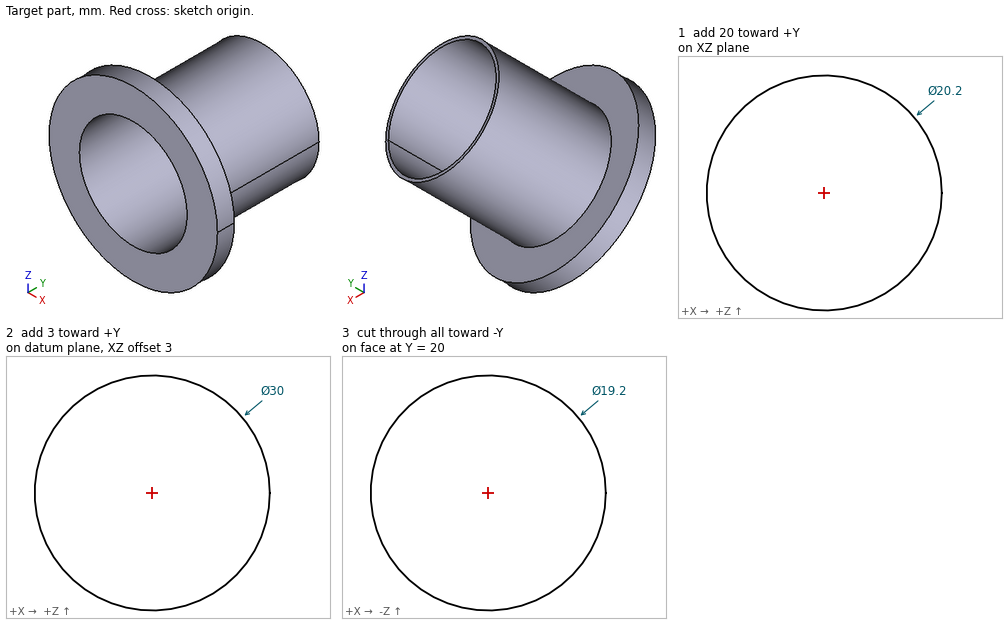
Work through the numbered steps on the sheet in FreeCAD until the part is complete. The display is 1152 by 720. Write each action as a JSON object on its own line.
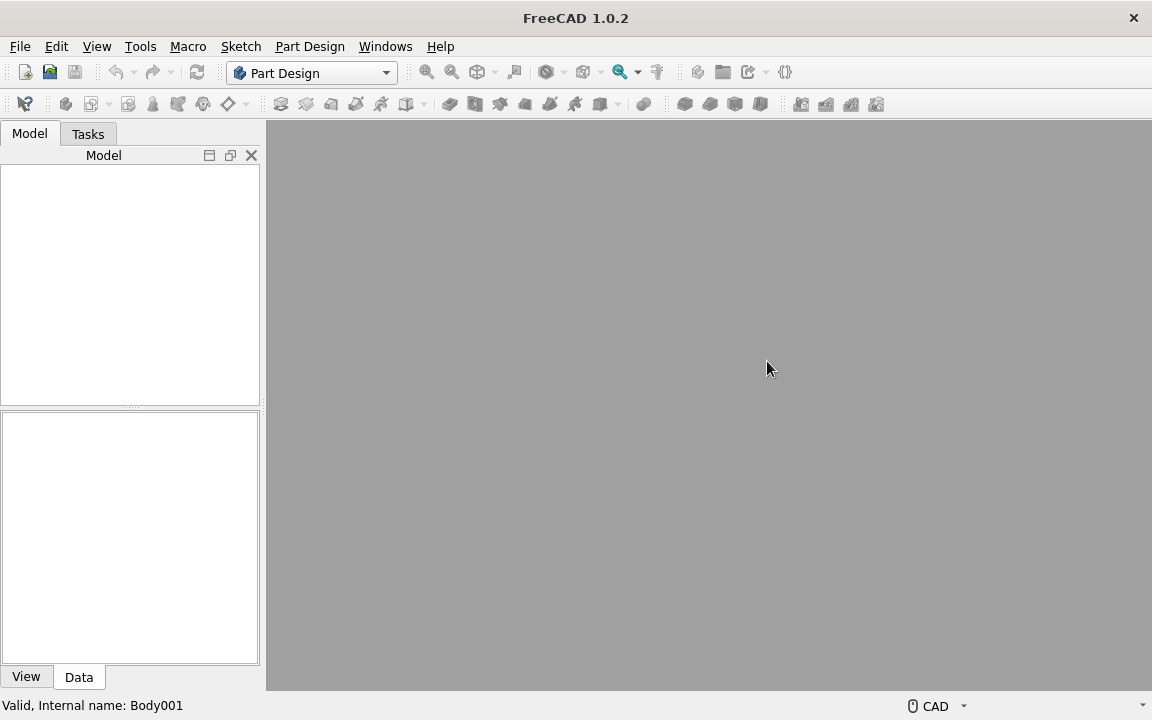
{"action": "key", "text": "ctrl+n"}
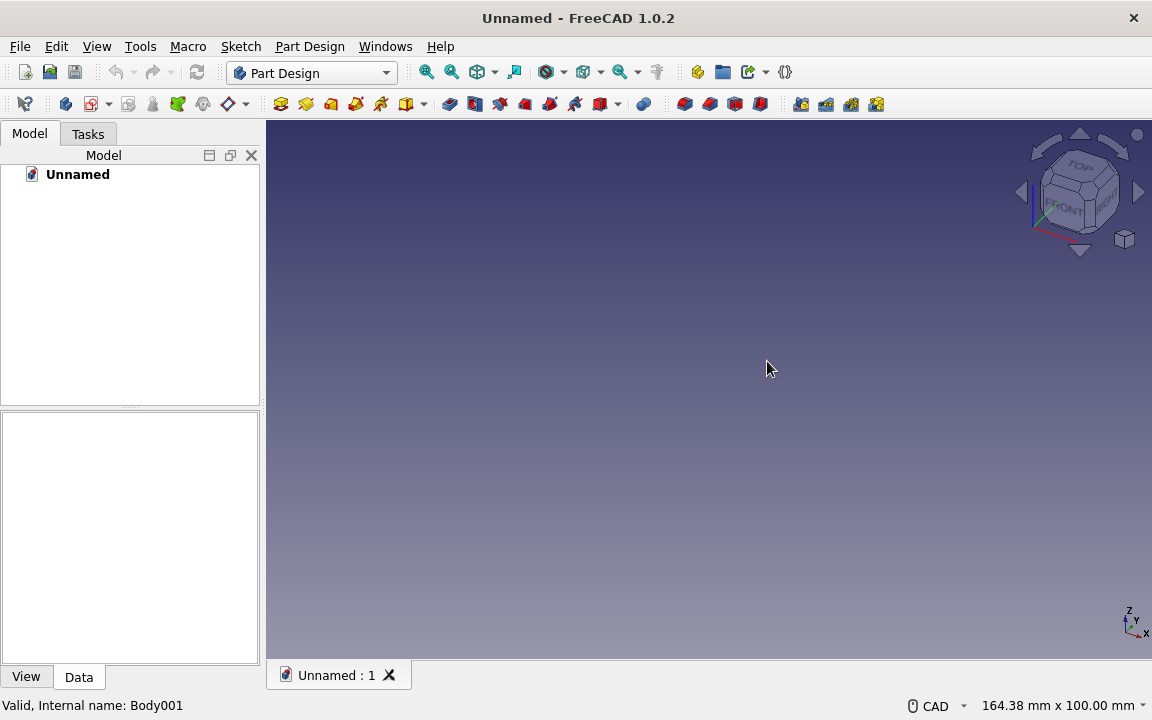
{"action": "left_click", "coordinate": [90, 104]}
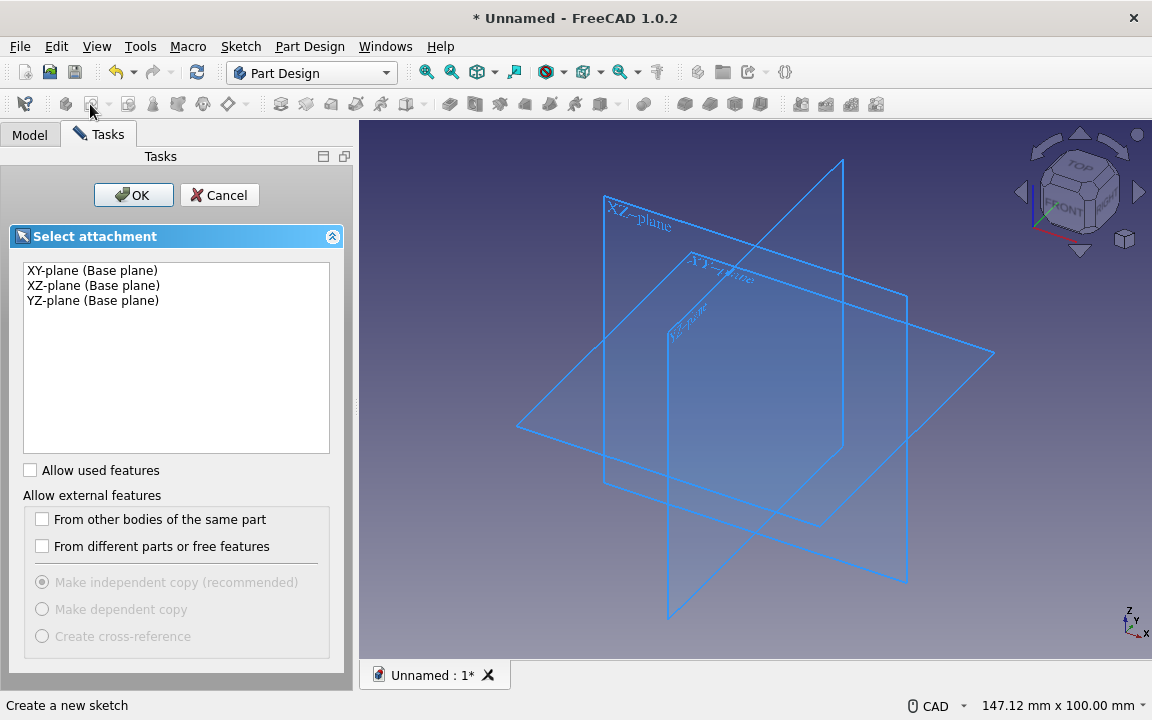
{"action": "left_click", "coordinate": [84, 286]}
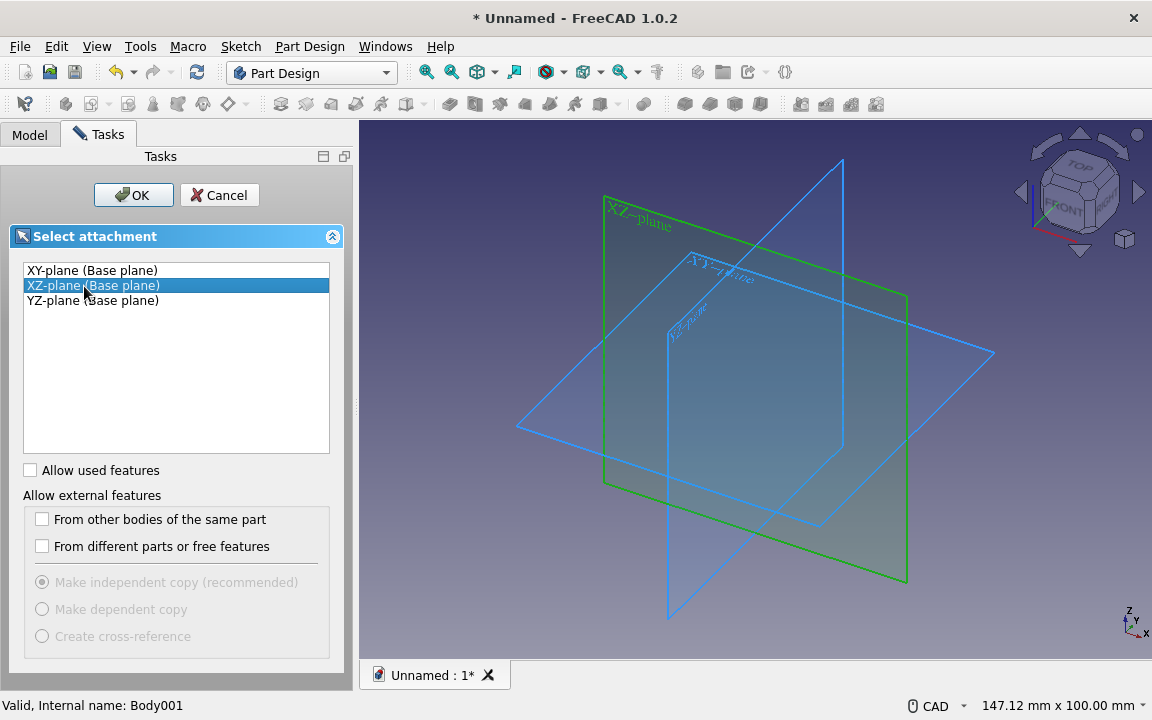
{"action": "left_click", "coordinate": [134, 195]}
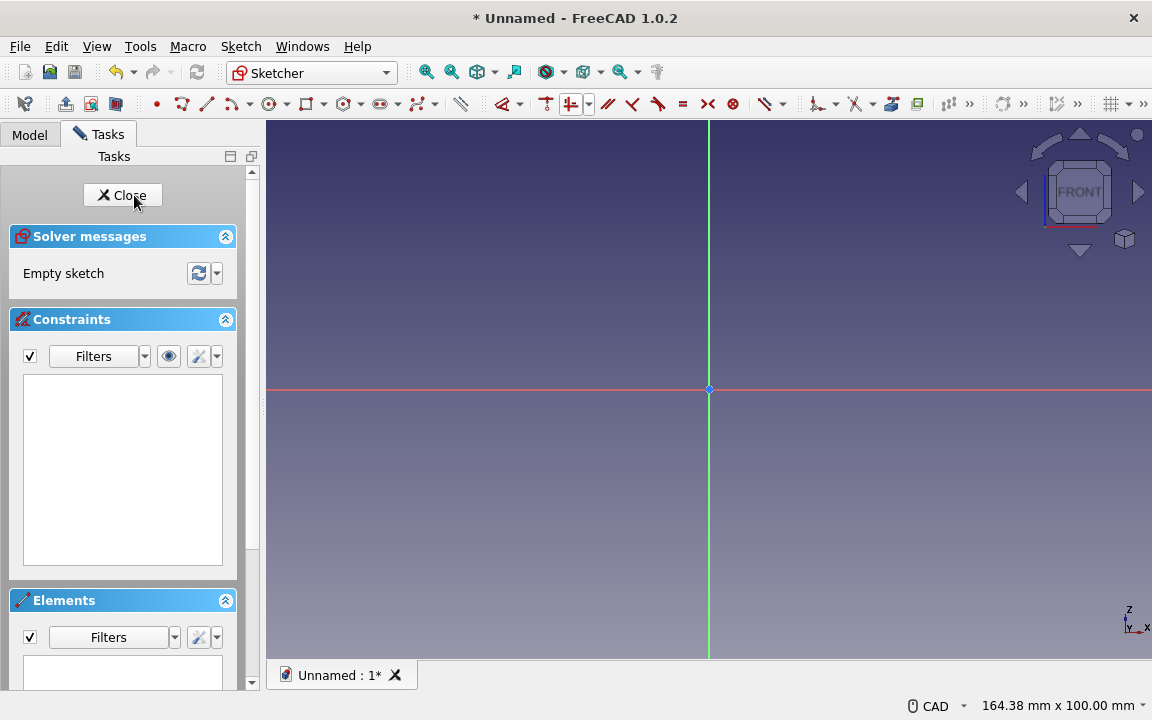
{"action": "scroll", "coordinate": [739, 390], "scroll_direction": "up", "scroll_amount": 6}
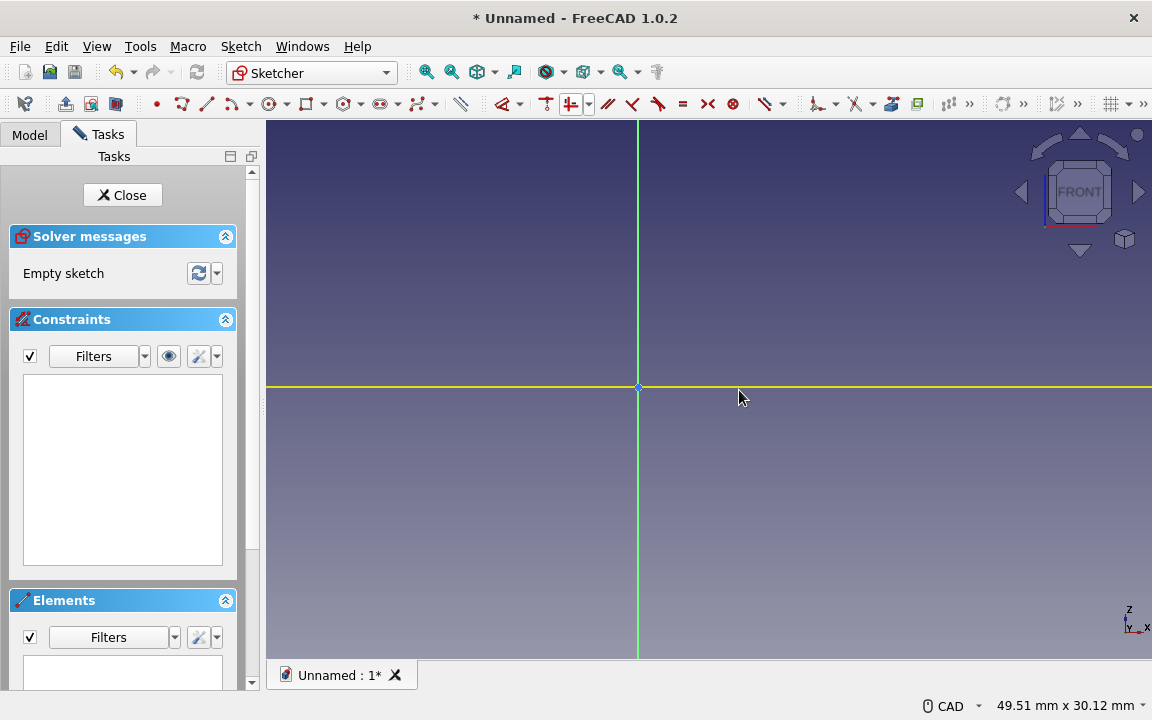
{"action": "key", "text": "g c"}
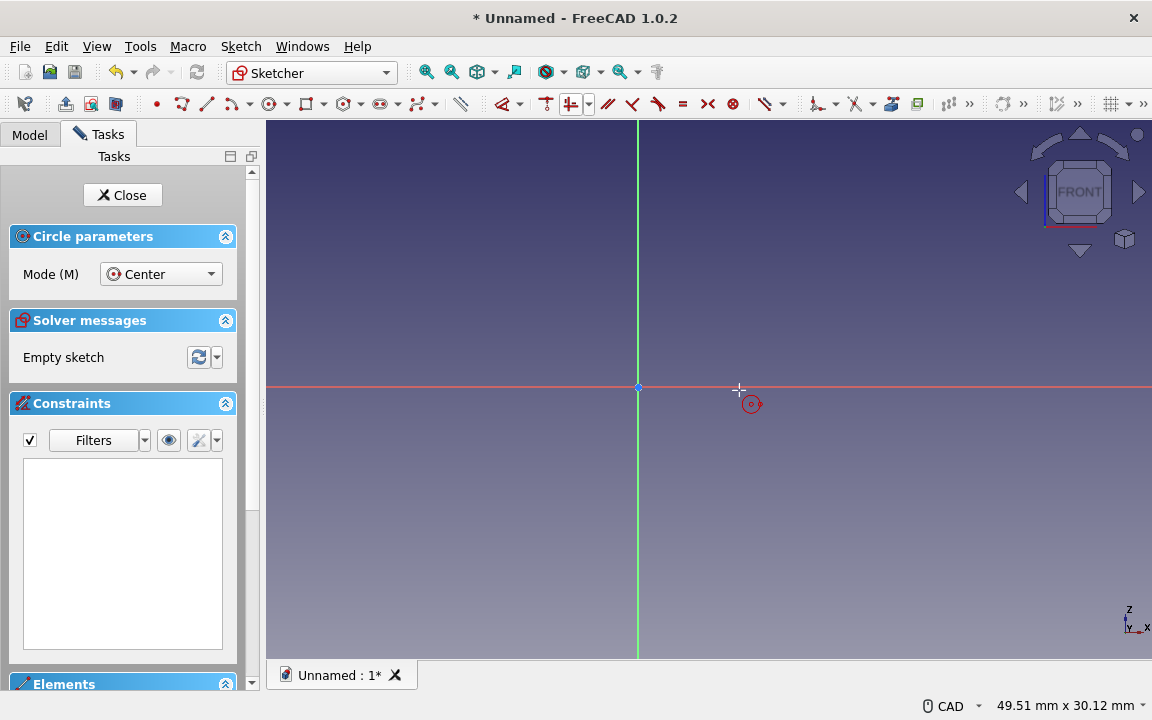
{"action": "left_click", "coordinate": [638, 387]}
{"action": "left_click", "coordinate": [766, 259]}
{"action": "key", "text": "Escape"}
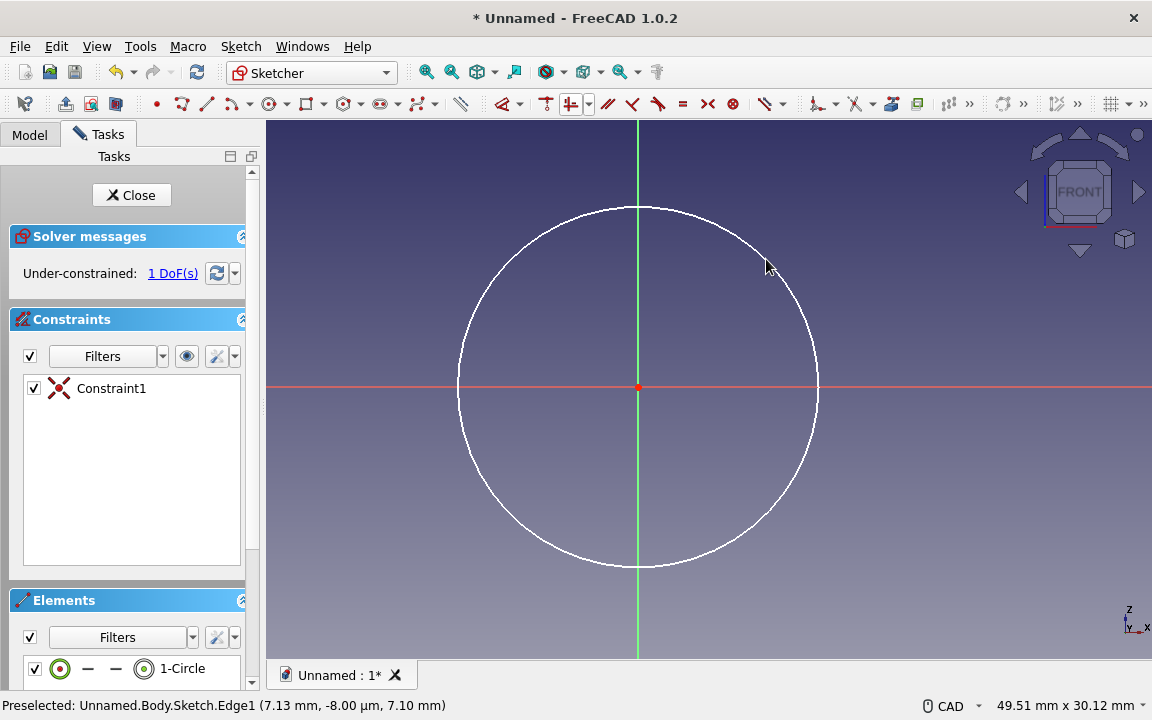
{"action": "key", "text": "d"}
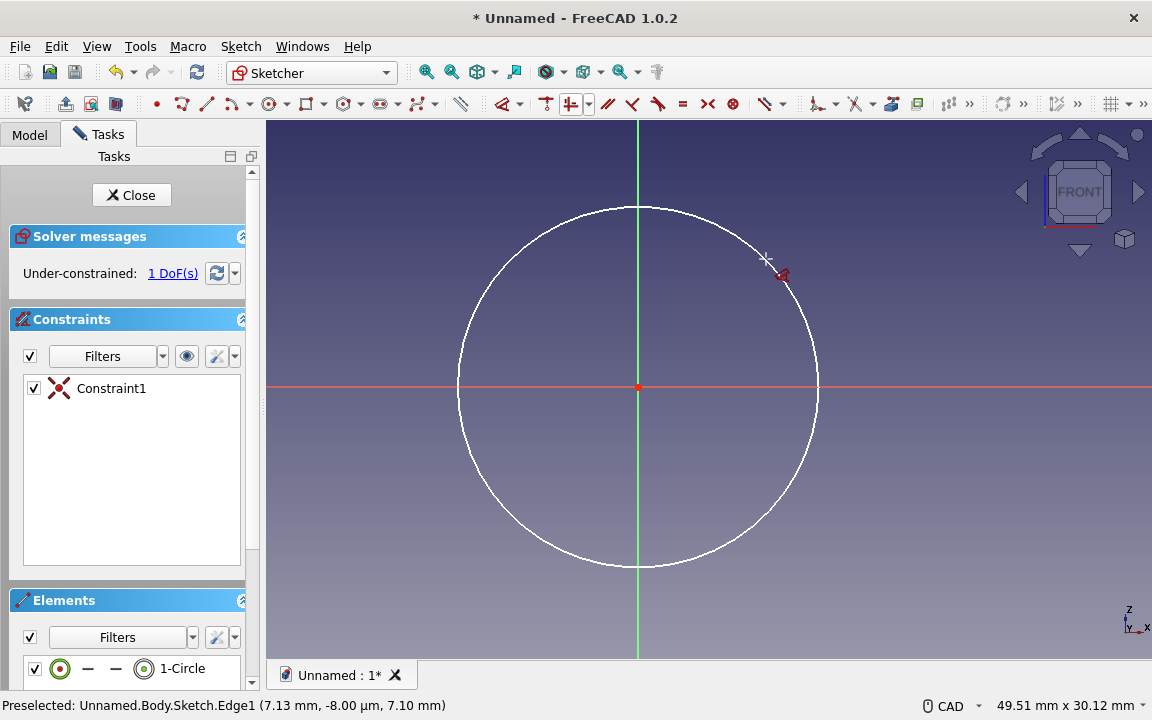
{"action": "left_click", "coordinate": [765, 259]}
{"action": "left_click", "coordinate": [788, 236]}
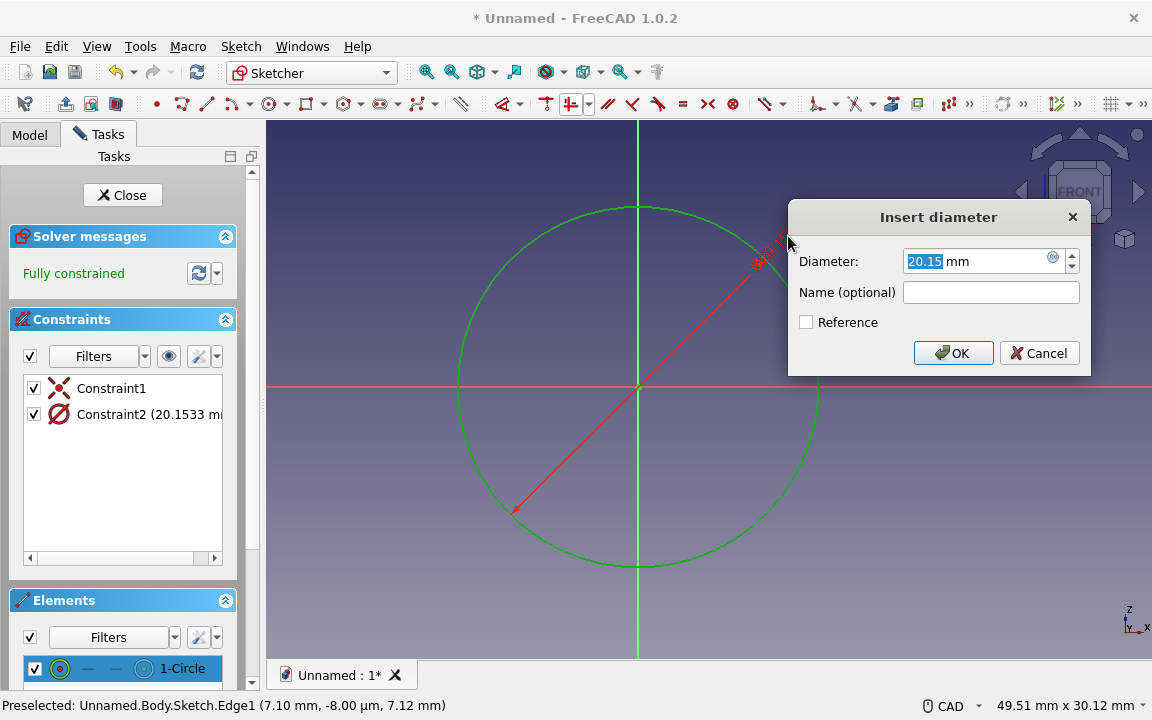
{"action": "type", "text": "20.2"}
{"action": "key", "text": "Return"}
{"action": "key", "text": "Escape"}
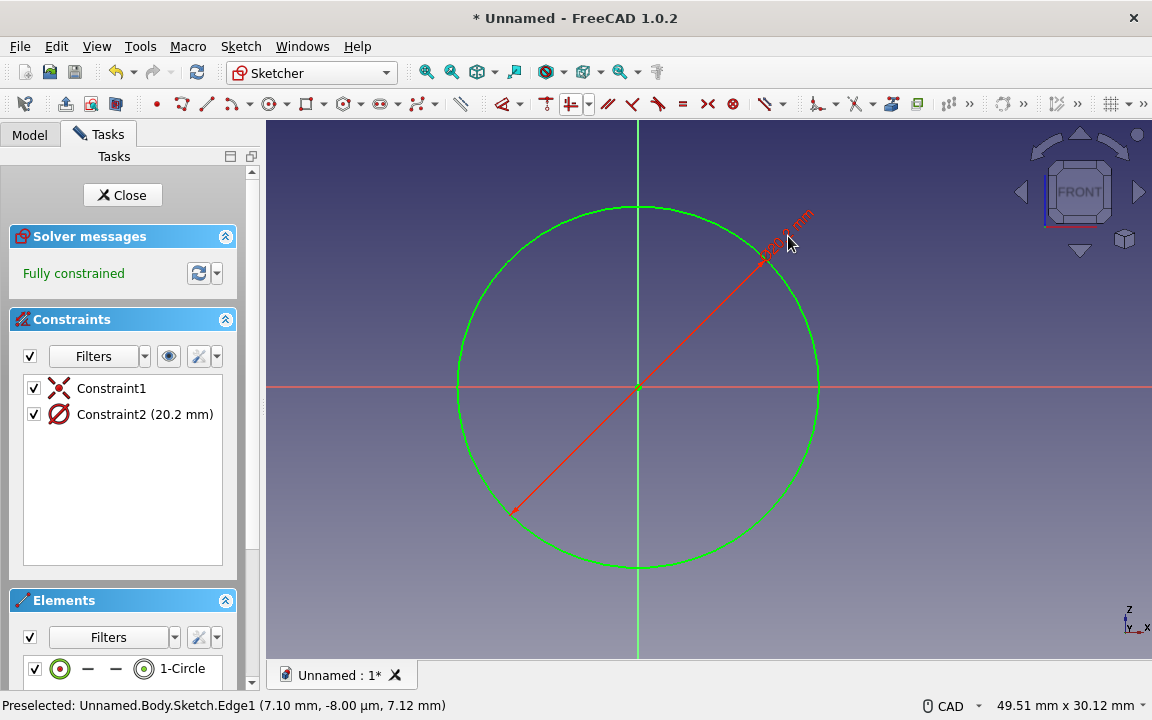
{"action": "left_click", "coordinate": [123, 195]}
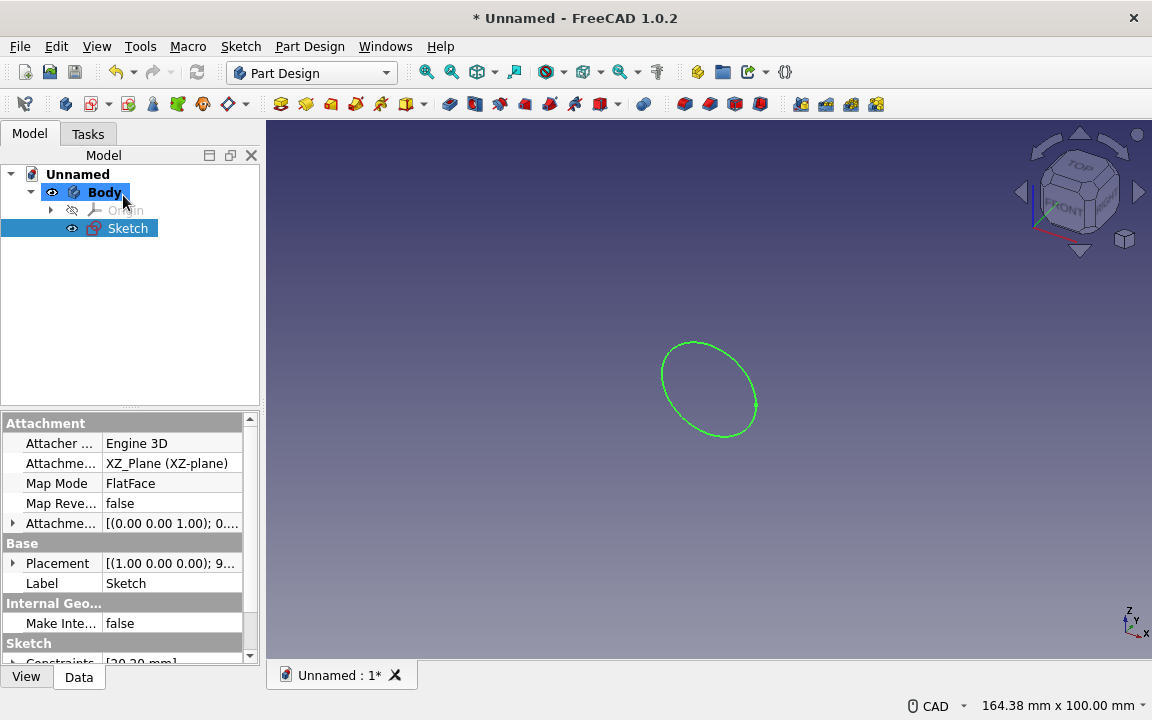
{"action": "left_click", "coordinate": [281, 104]}